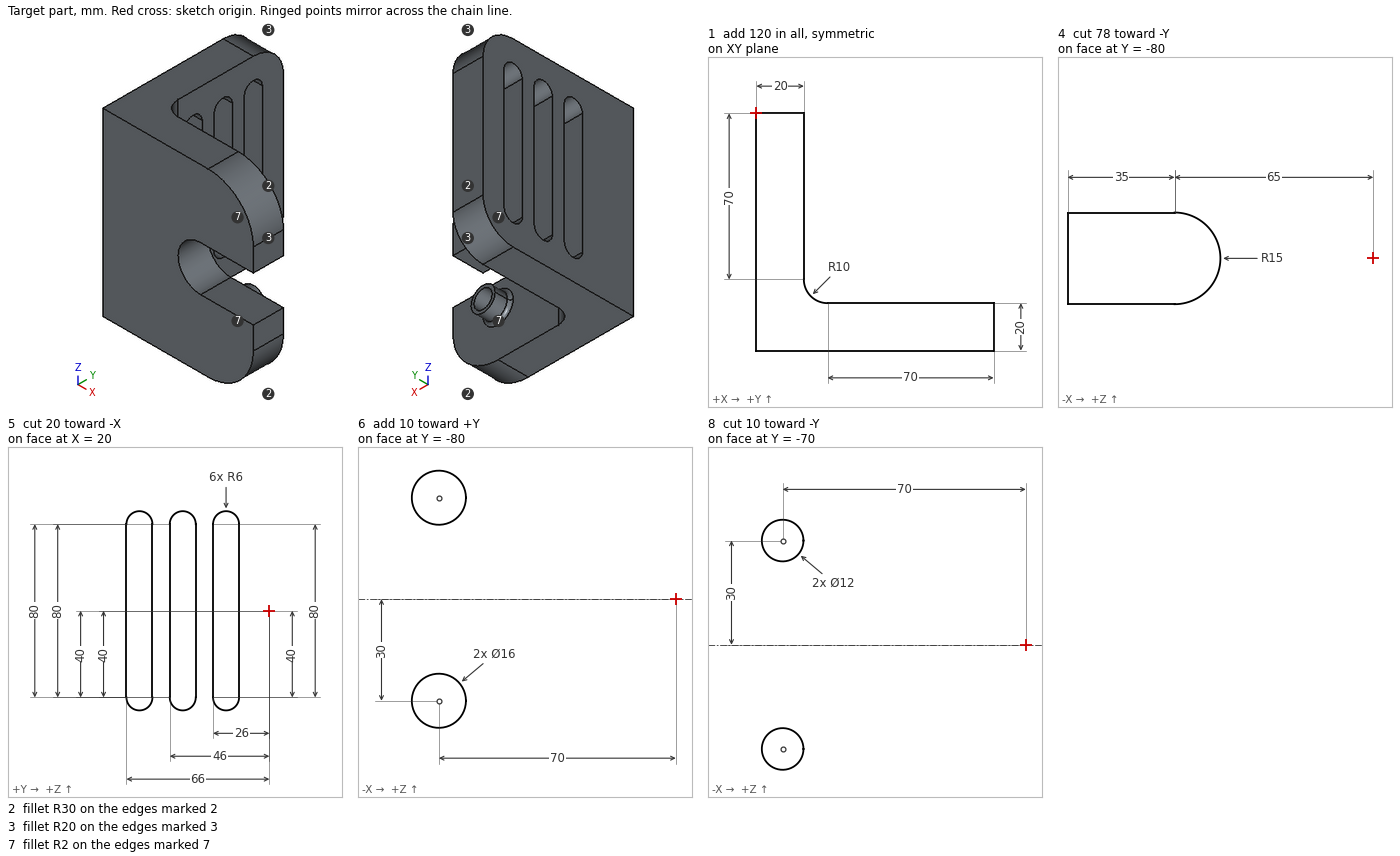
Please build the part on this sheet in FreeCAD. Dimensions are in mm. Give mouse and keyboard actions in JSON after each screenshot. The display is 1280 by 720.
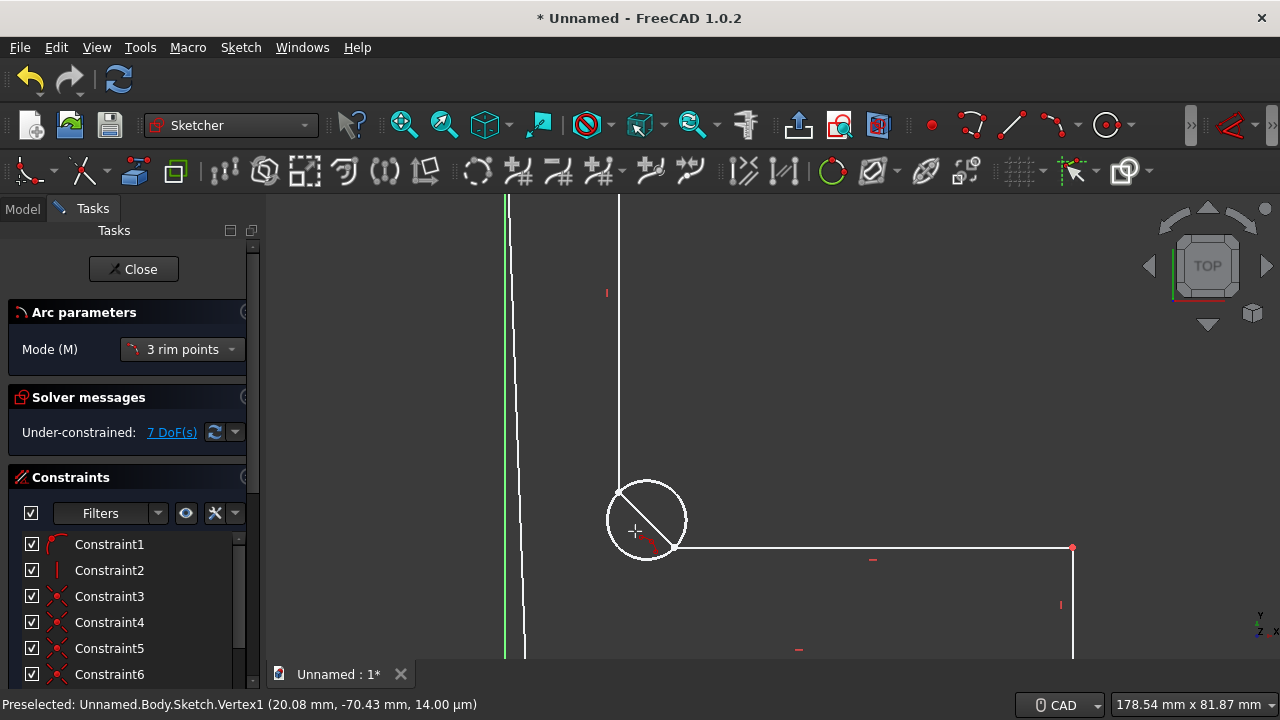
{"action": "left_click", "coordinate": [635, 530]}
{"action": "key", "text": "Escape"}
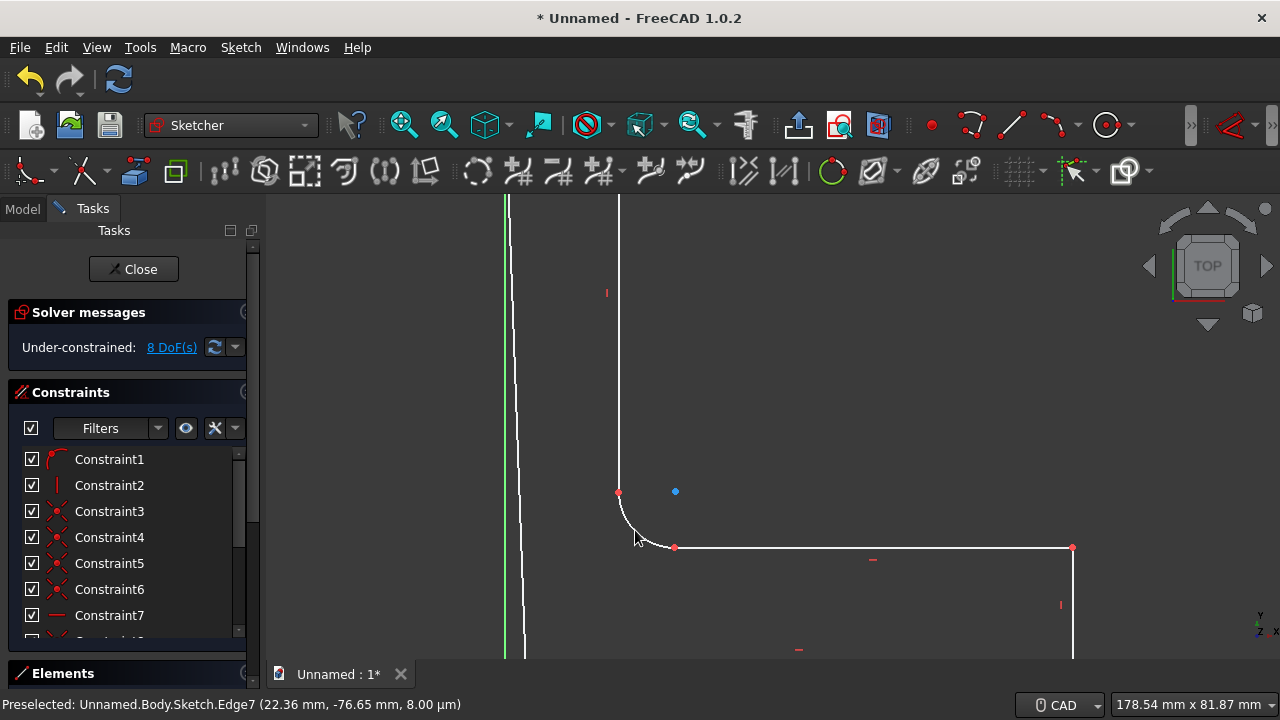
{"action": "left_click", "coordinate": [619, 372]}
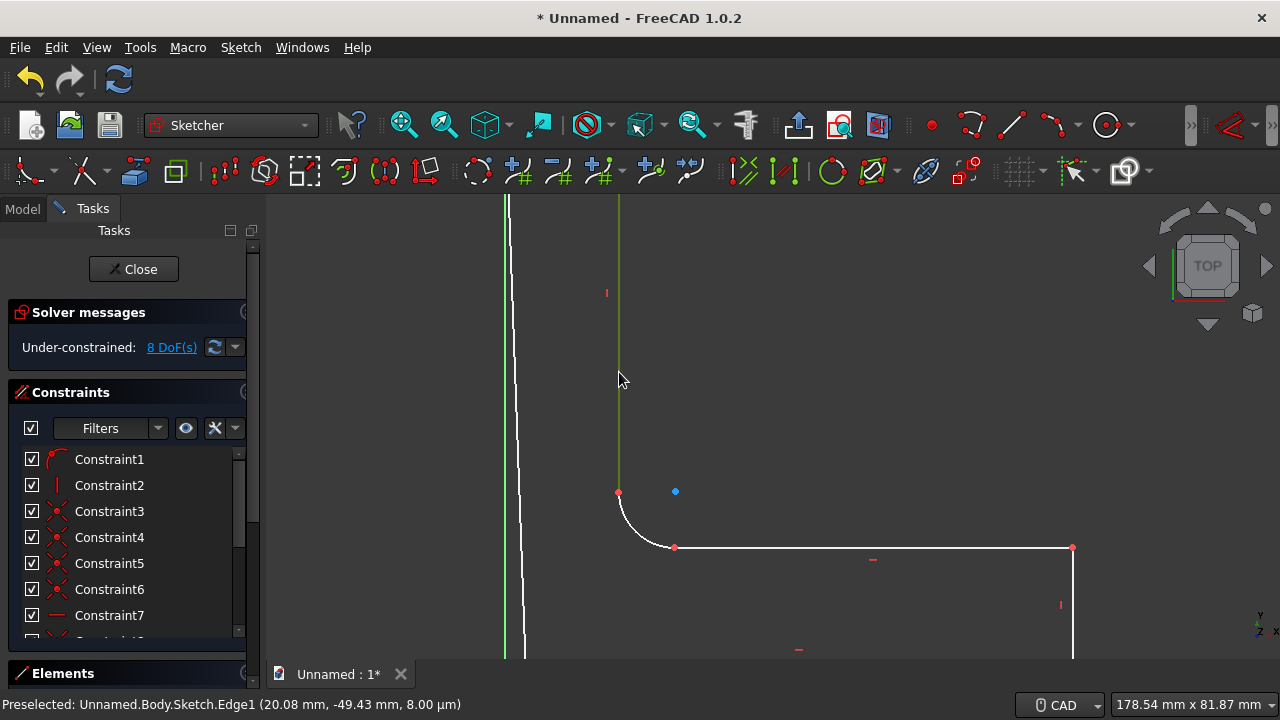
{"action": "left_click", "coordinate": [625, 517]}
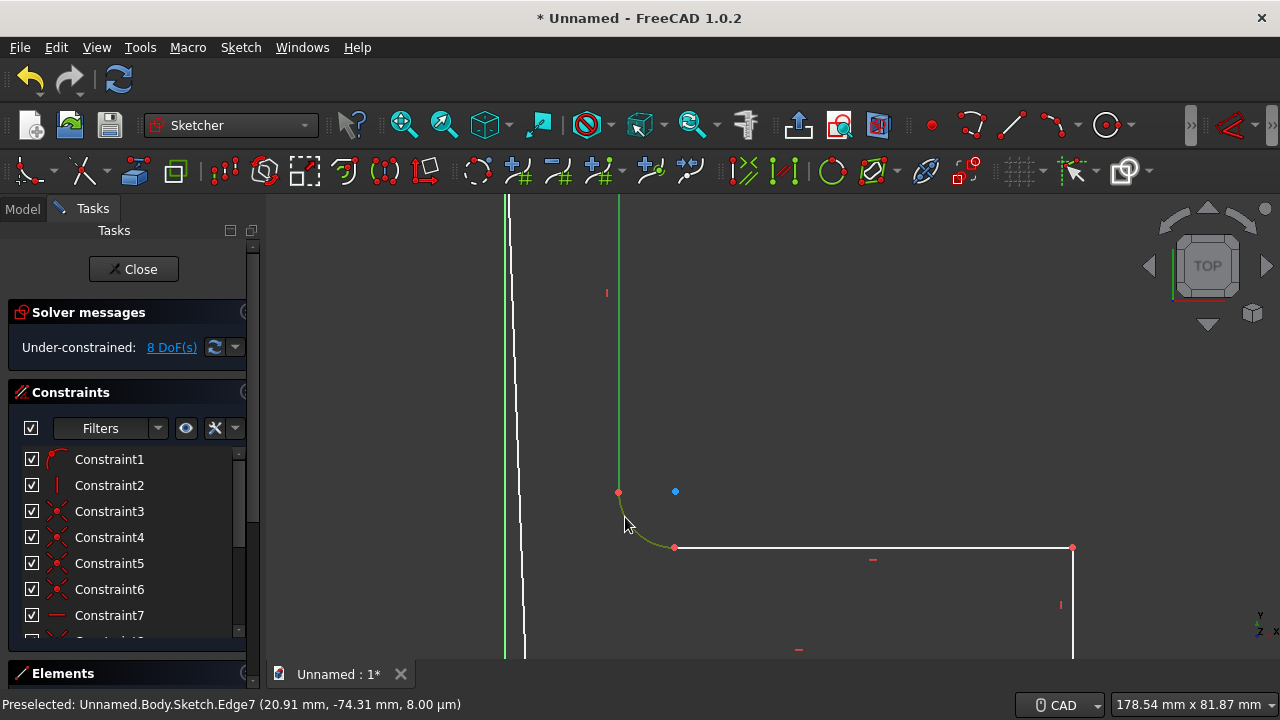
{"action": "key", "text": "t"}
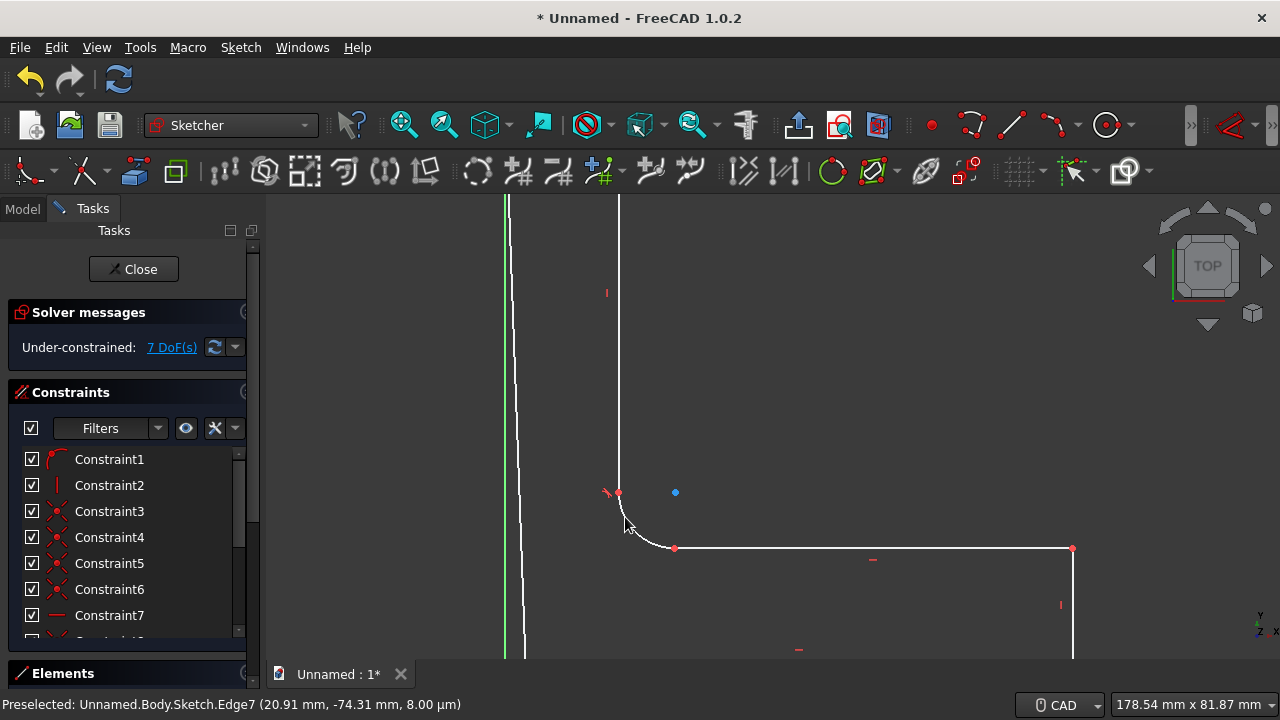
{"action": "left_click", "coordinate": [953, 548]}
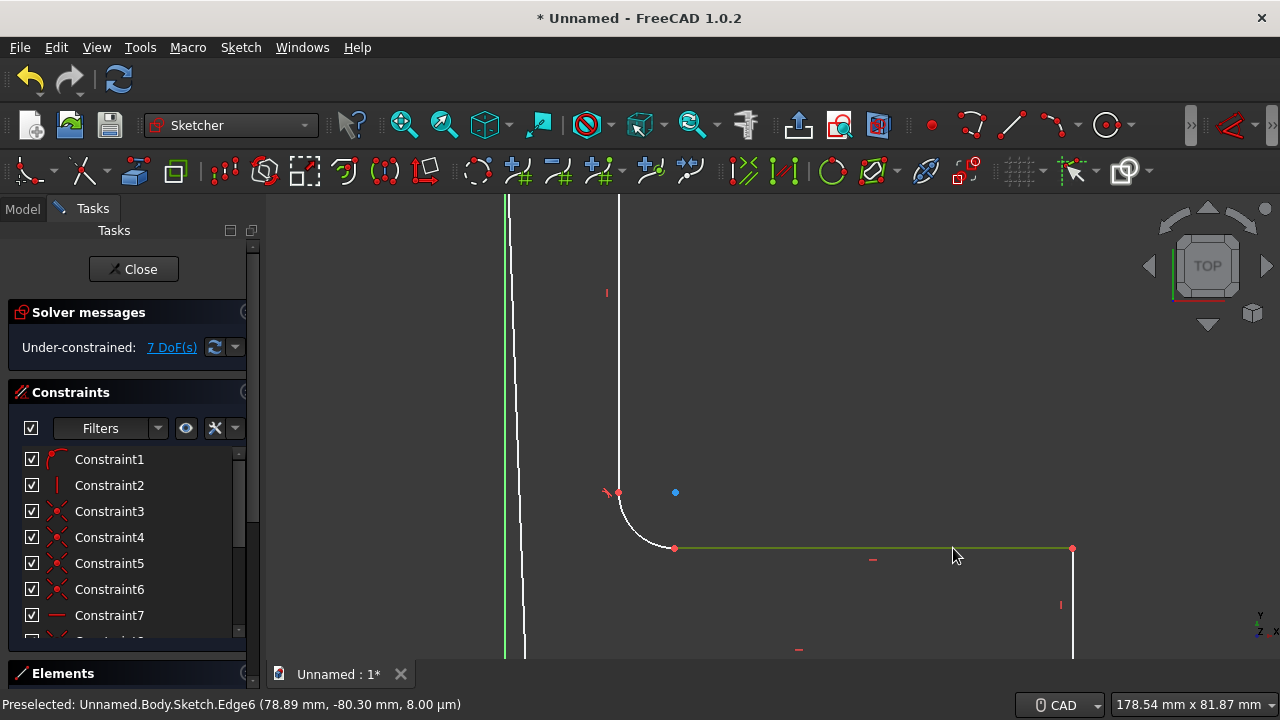
{"action": "left_click", "coordinate": [625, 517]}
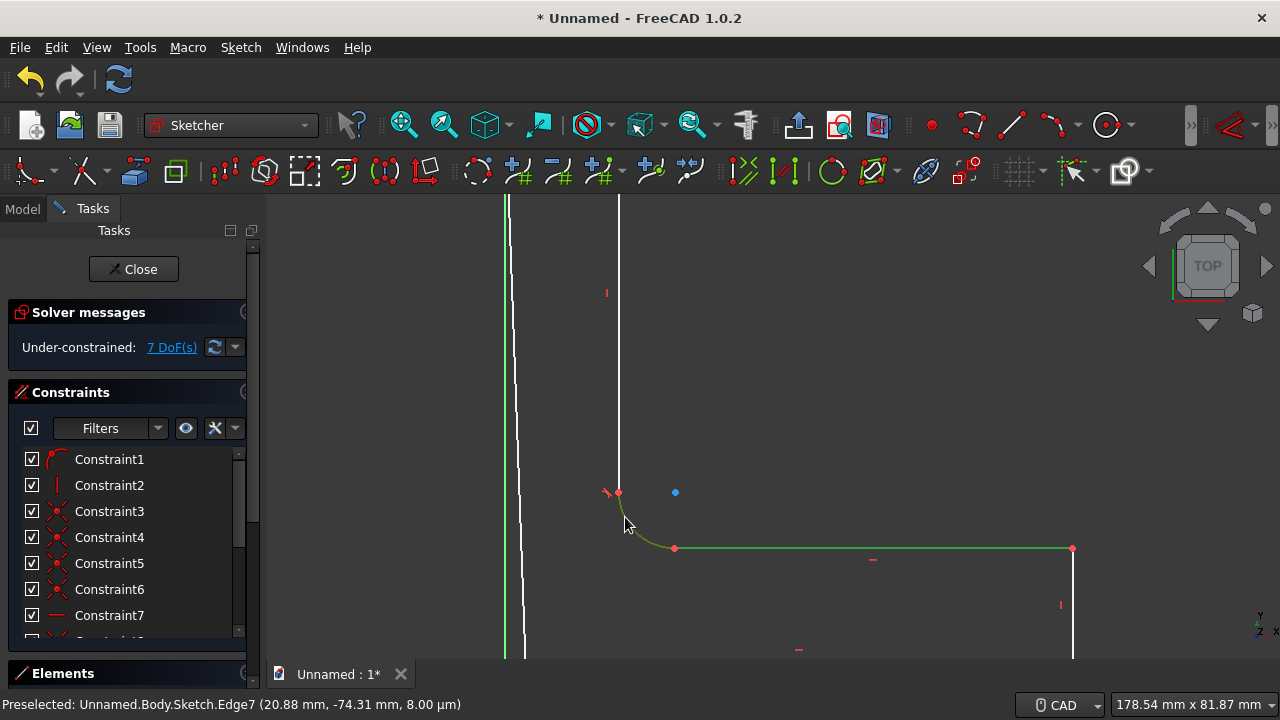
{"action": "key", "text": "t"}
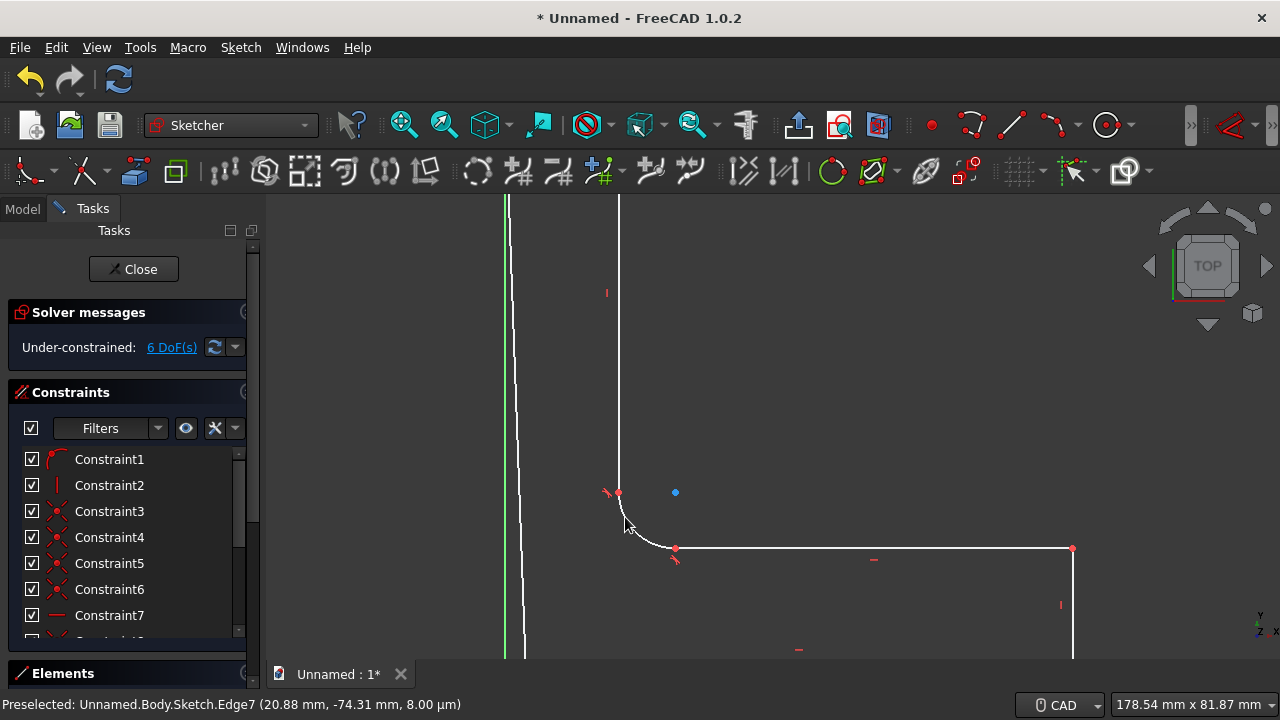
{"action": "left_click", "coordinate": [519, 491]}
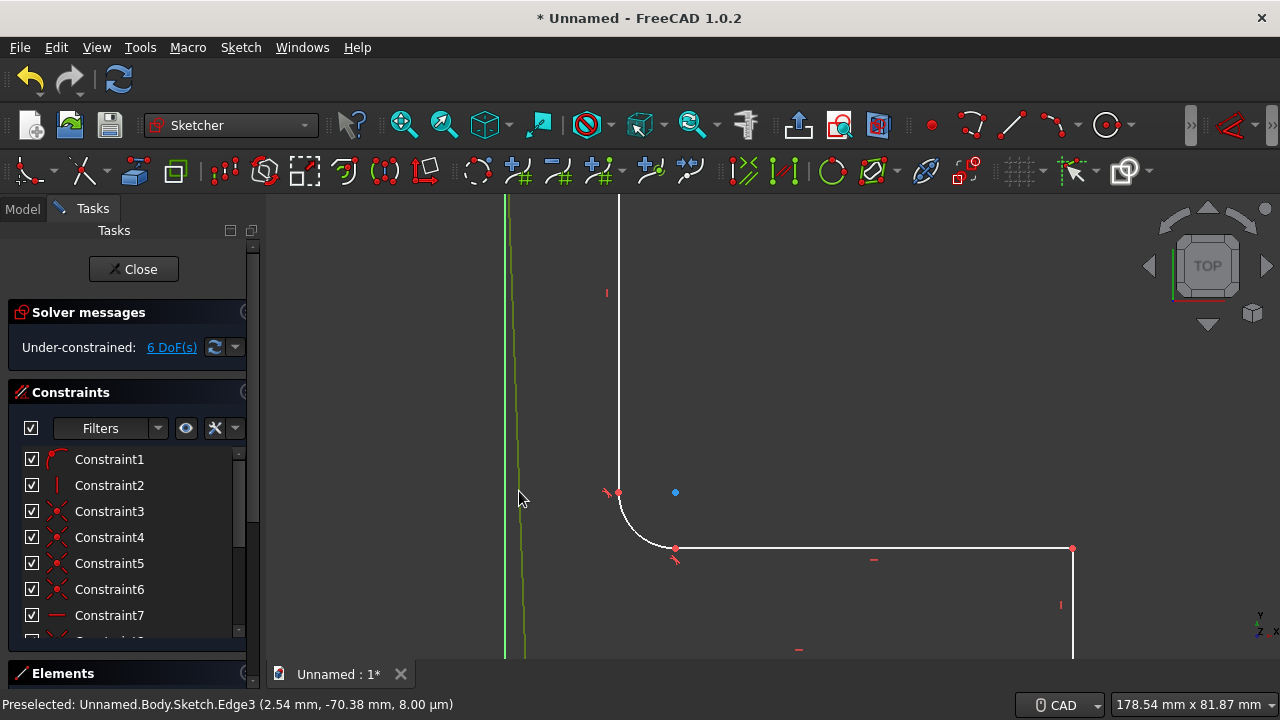
{"action": "key", "text": "v"}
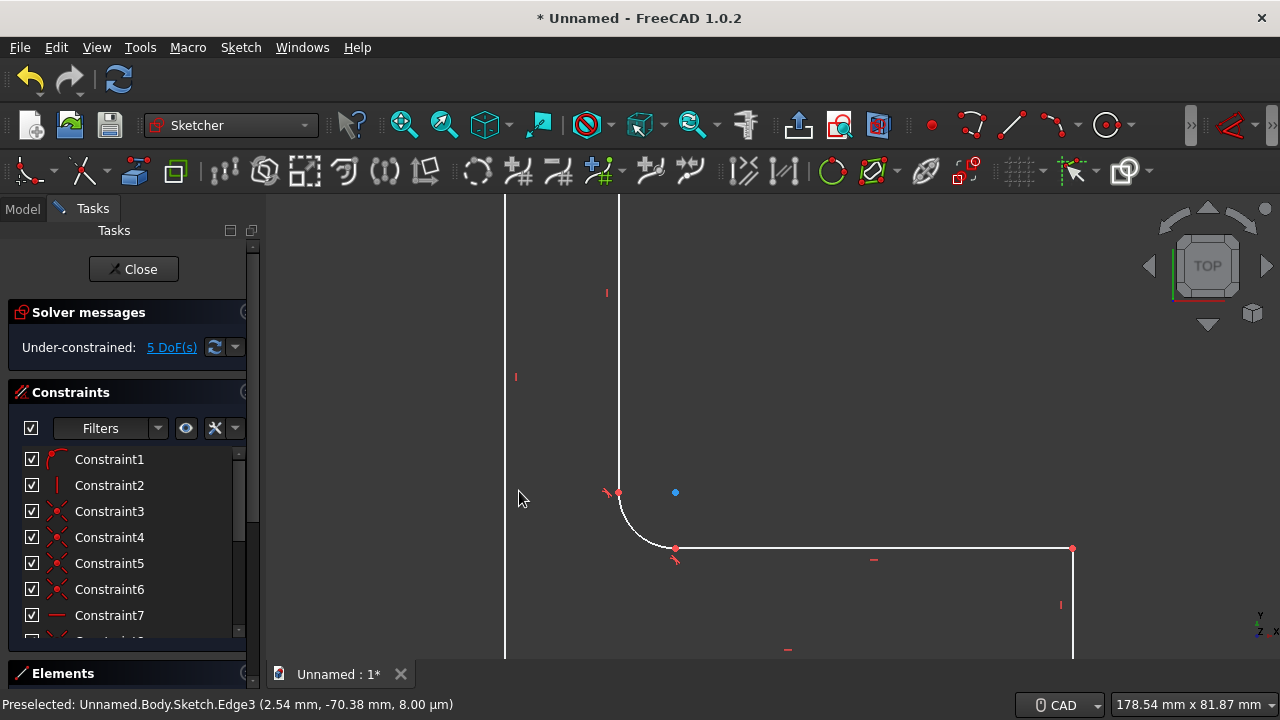
{"action": "left_click", "coordinate": [1230, 126]}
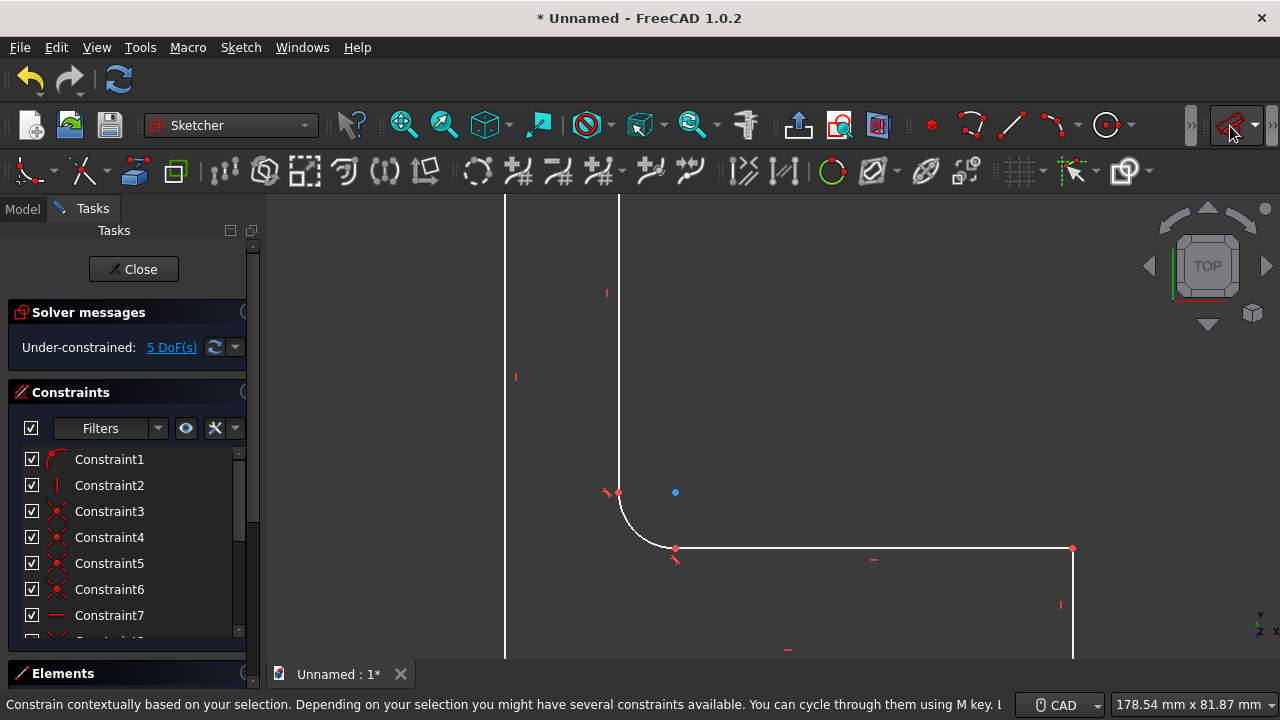
{"action": "left_click", "coordinate": [625, 518]}
{"action": "left_click", "coordinate": [597, 533]}